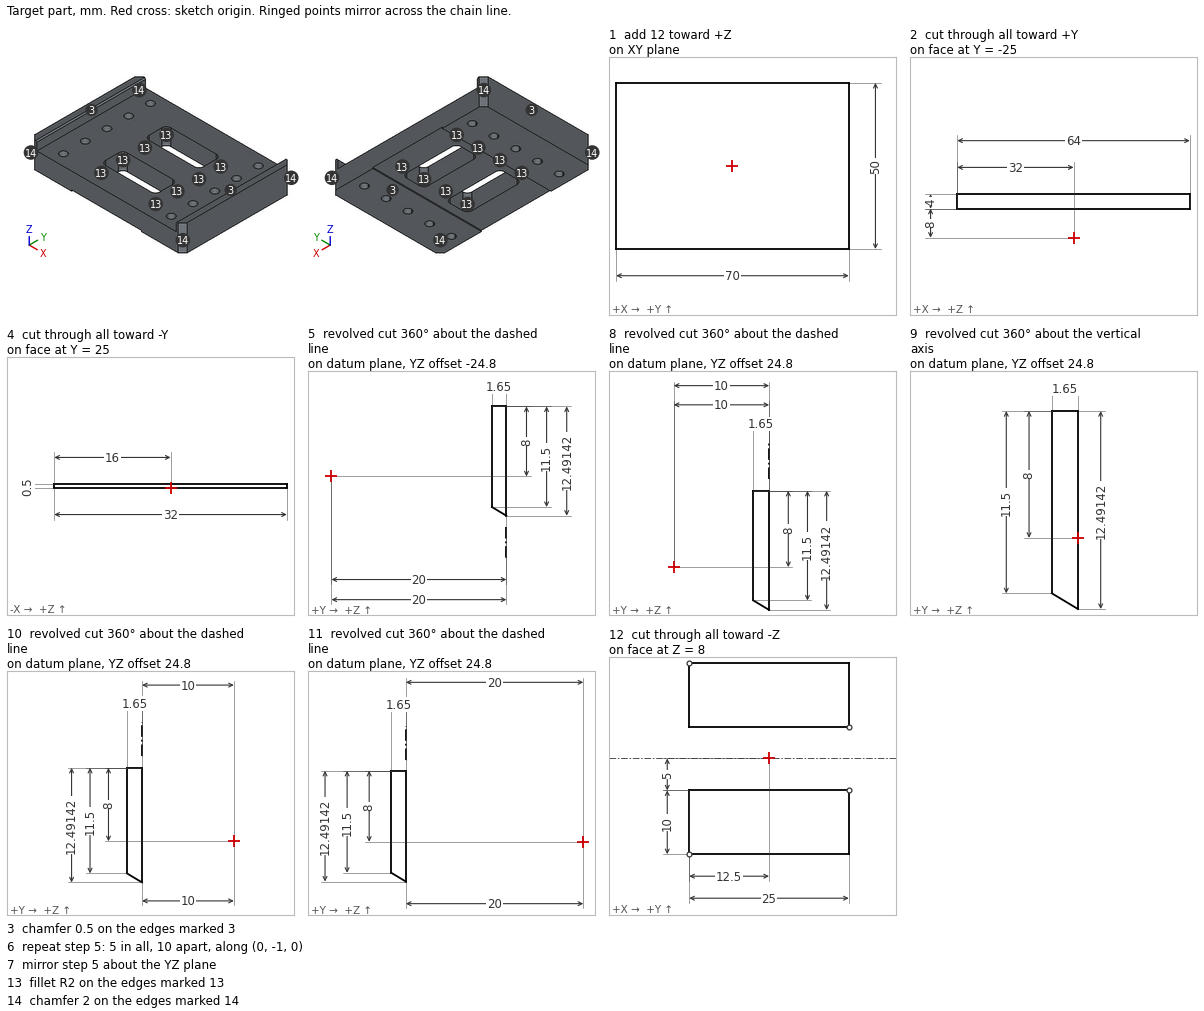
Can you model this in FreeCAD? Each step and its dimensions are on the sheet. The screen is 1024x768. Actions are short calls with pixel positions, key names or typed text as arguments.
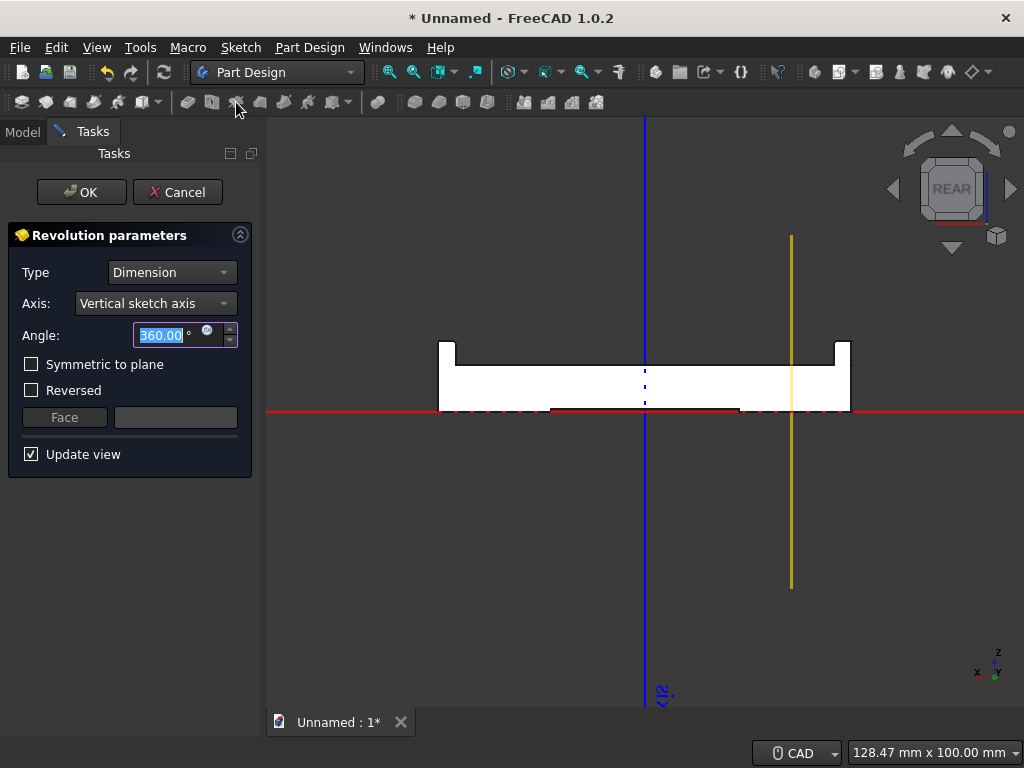
click(156, 304)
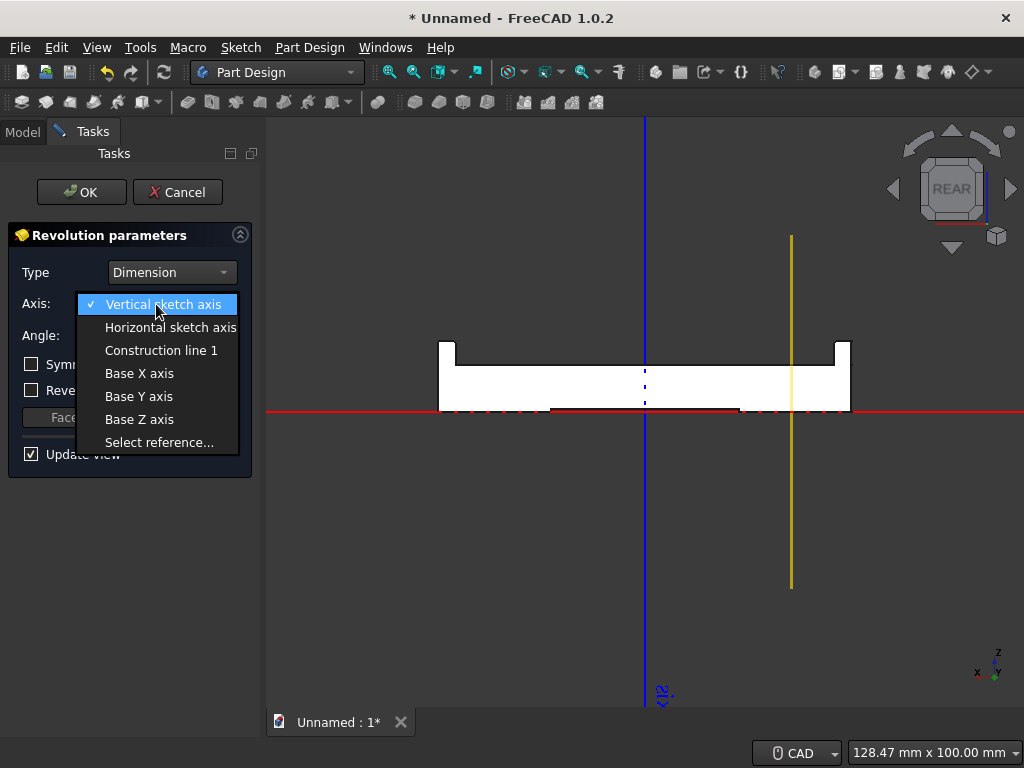
click(156, 350)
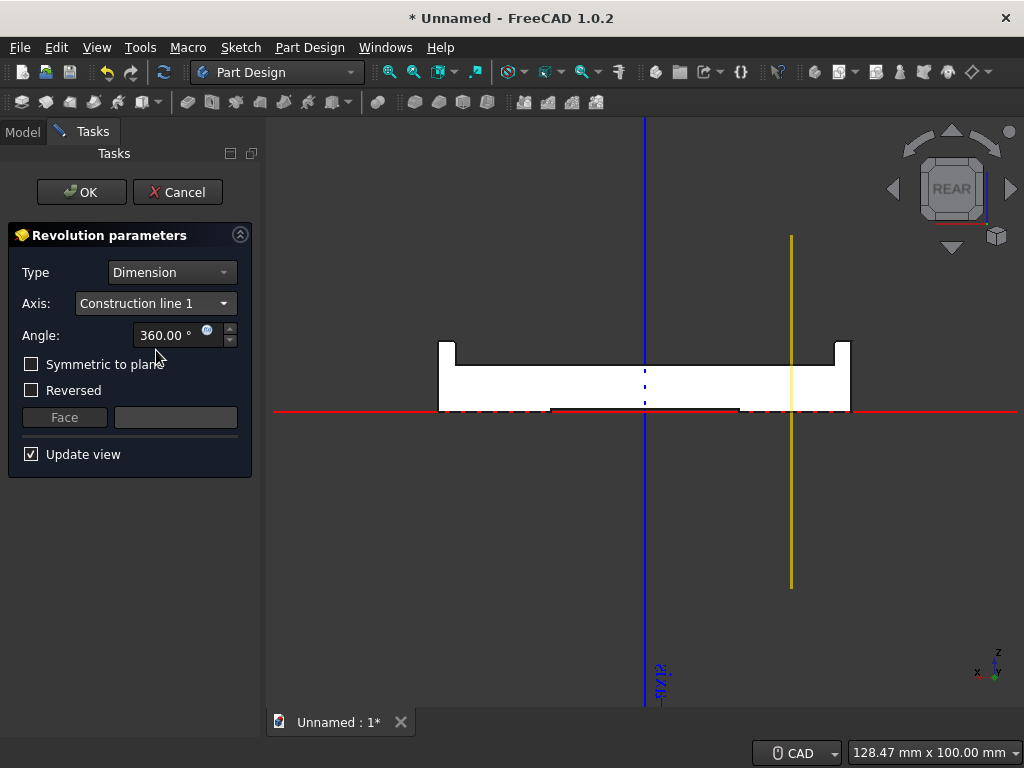
click(82, 192)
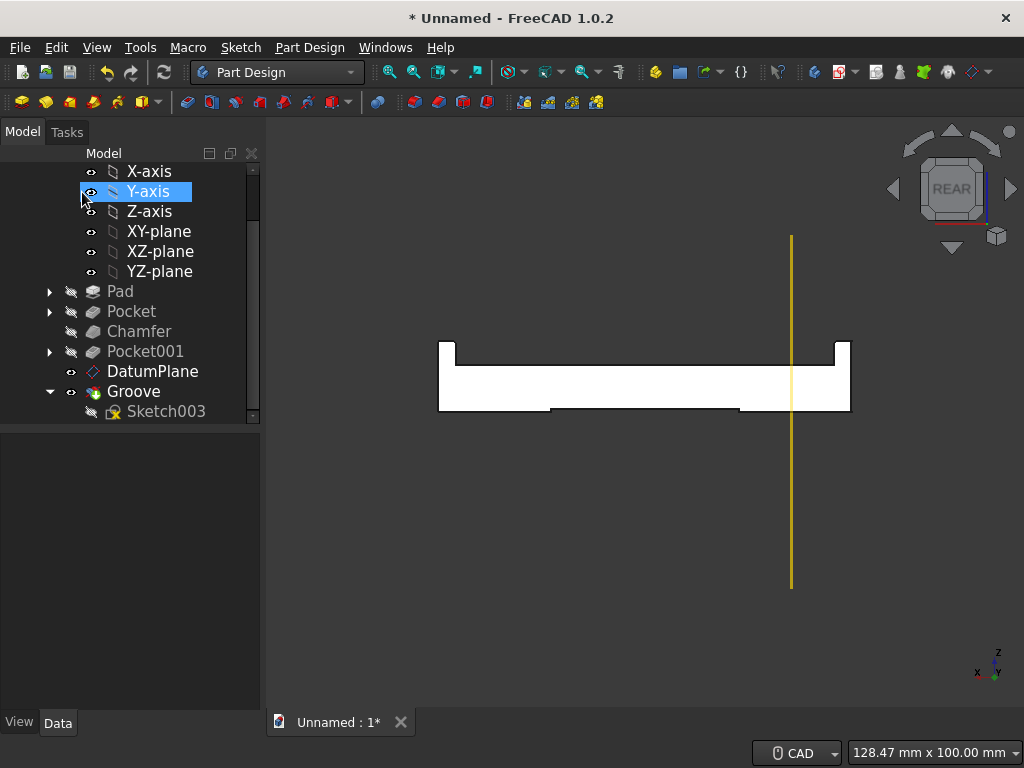
click(116, 372)
key(space)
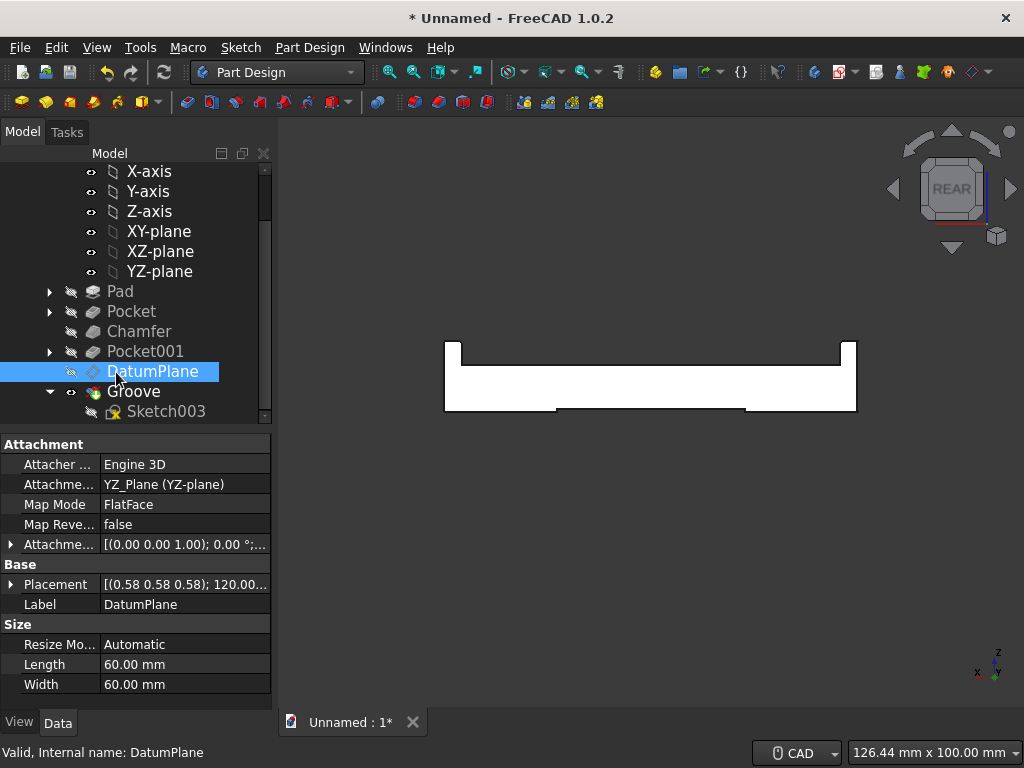
click(116, 392)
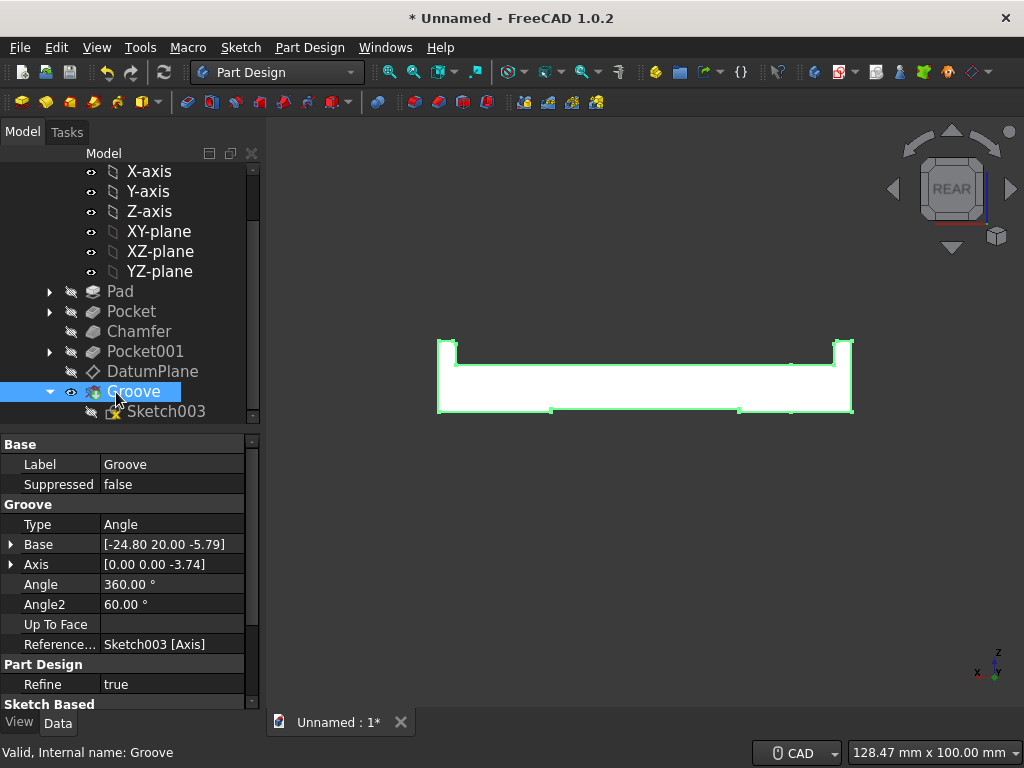
click(548, 102)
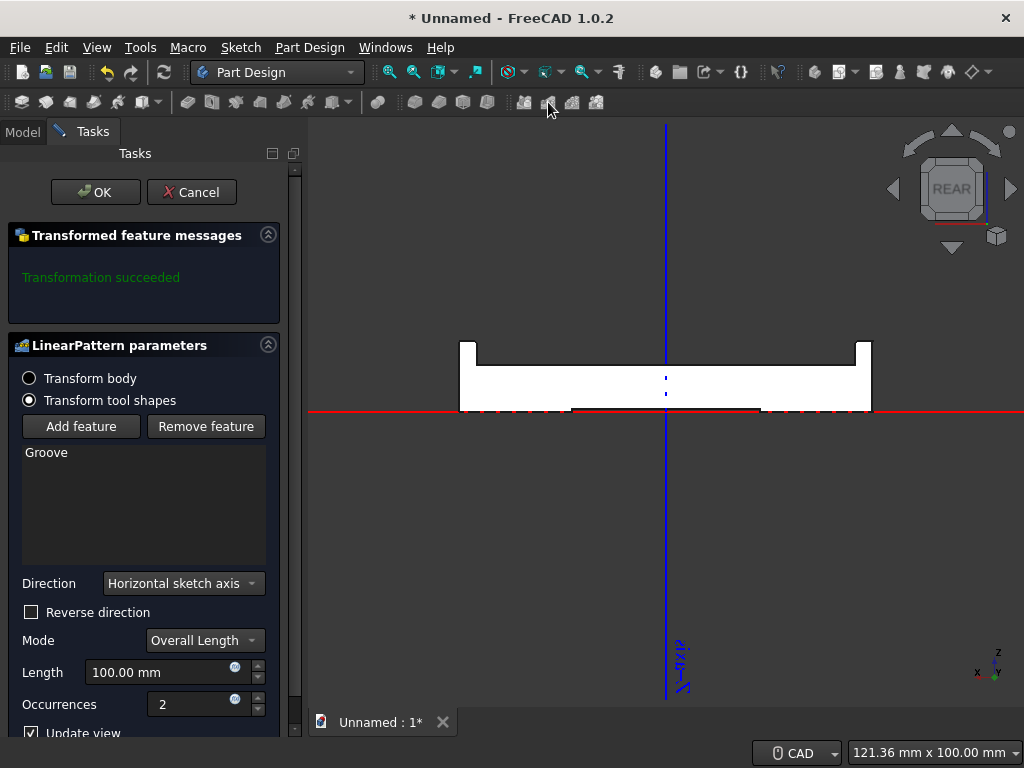
click(184, 584)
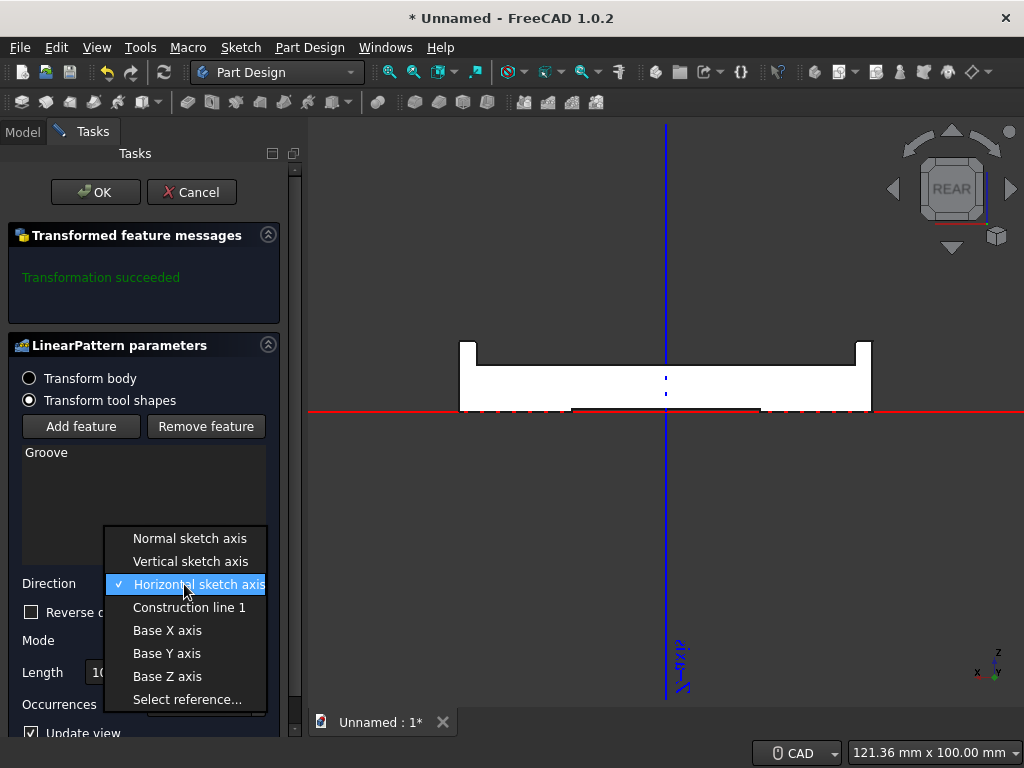
click(184, 654)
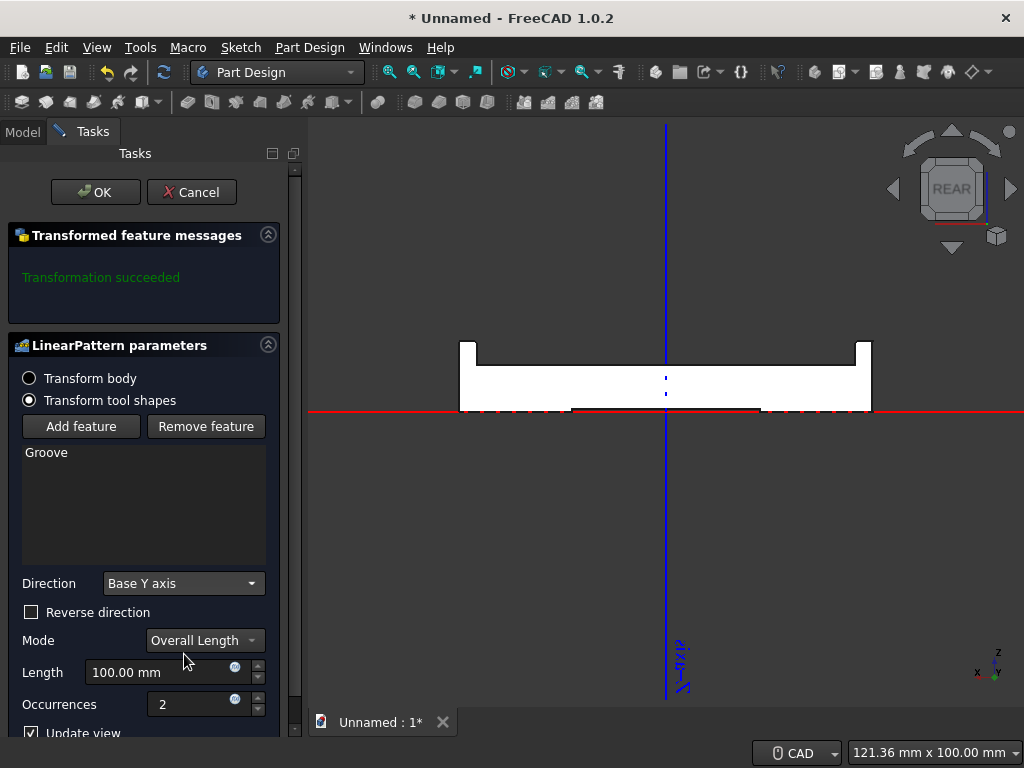
click(206, 640)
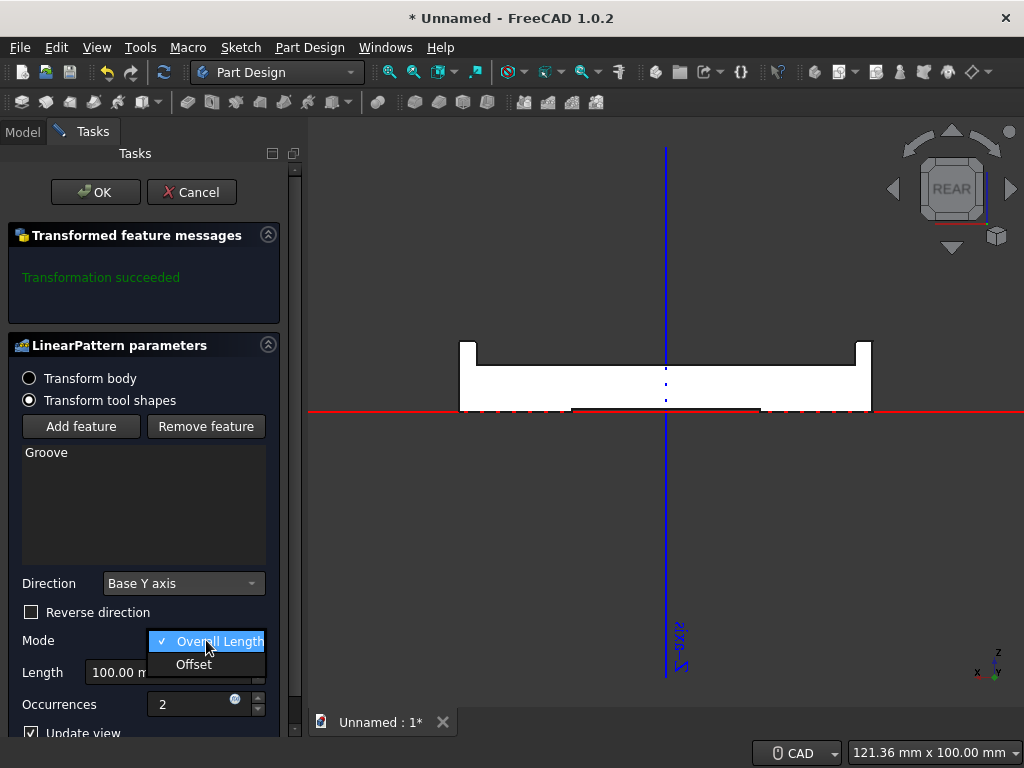
click(206, 664)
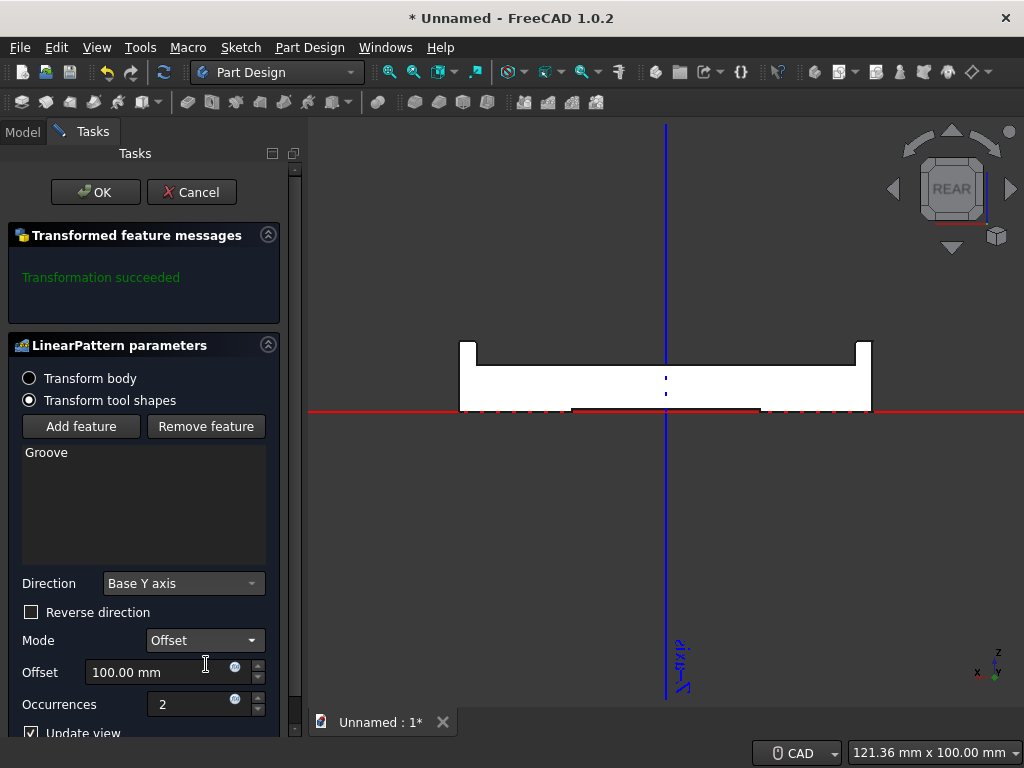
triple_click(168, 672)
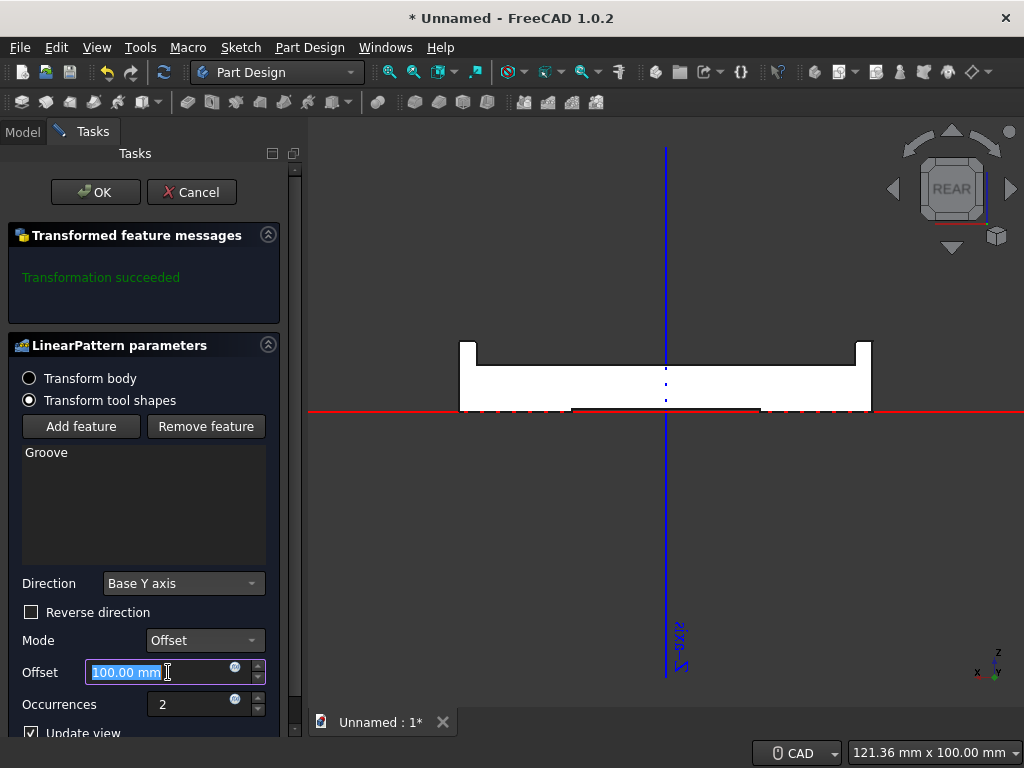
text(10)
key(Tab)